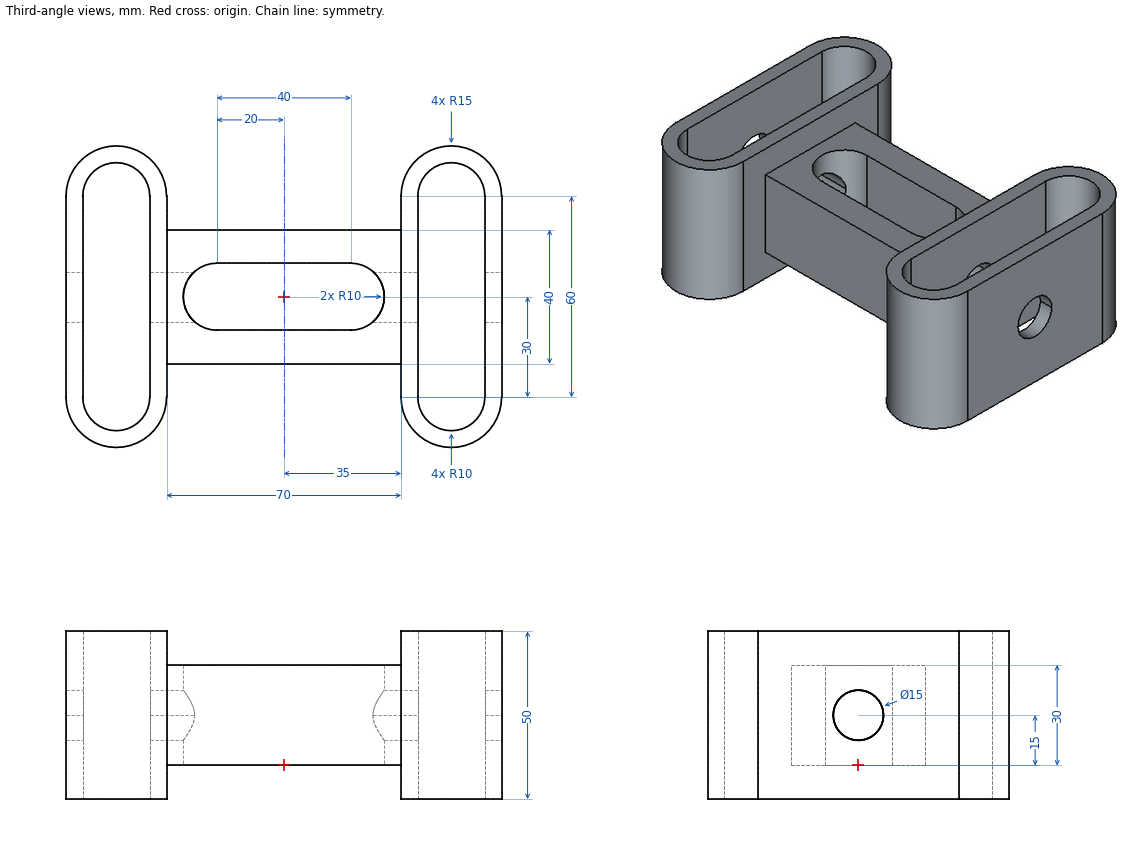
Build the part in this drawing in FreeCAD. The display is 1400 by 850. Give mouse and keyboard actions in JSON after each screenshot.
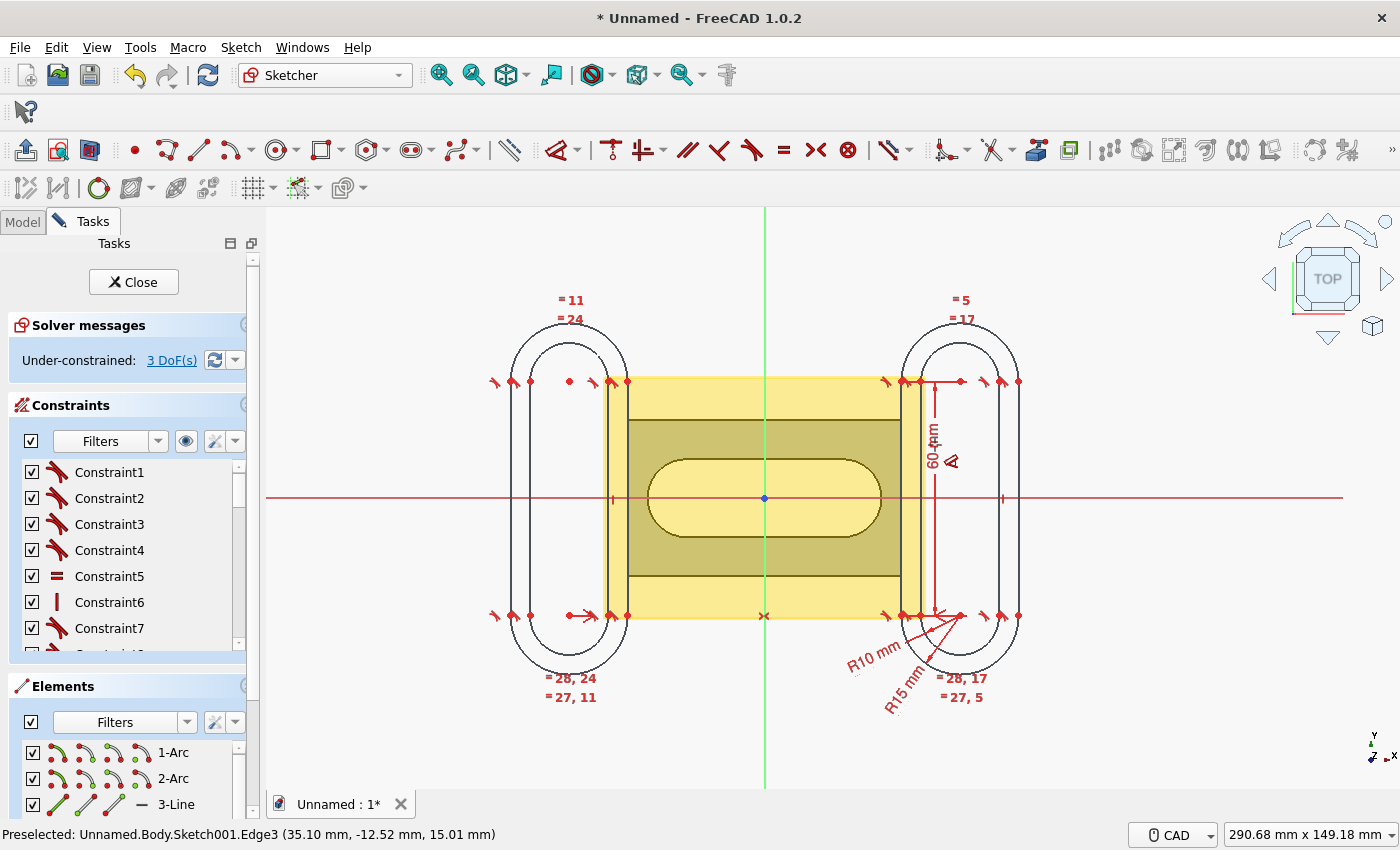
{"action": "left_click", "coordinate": [511, 546]}
{"action": "left_click", "coordinate": [477, 445]}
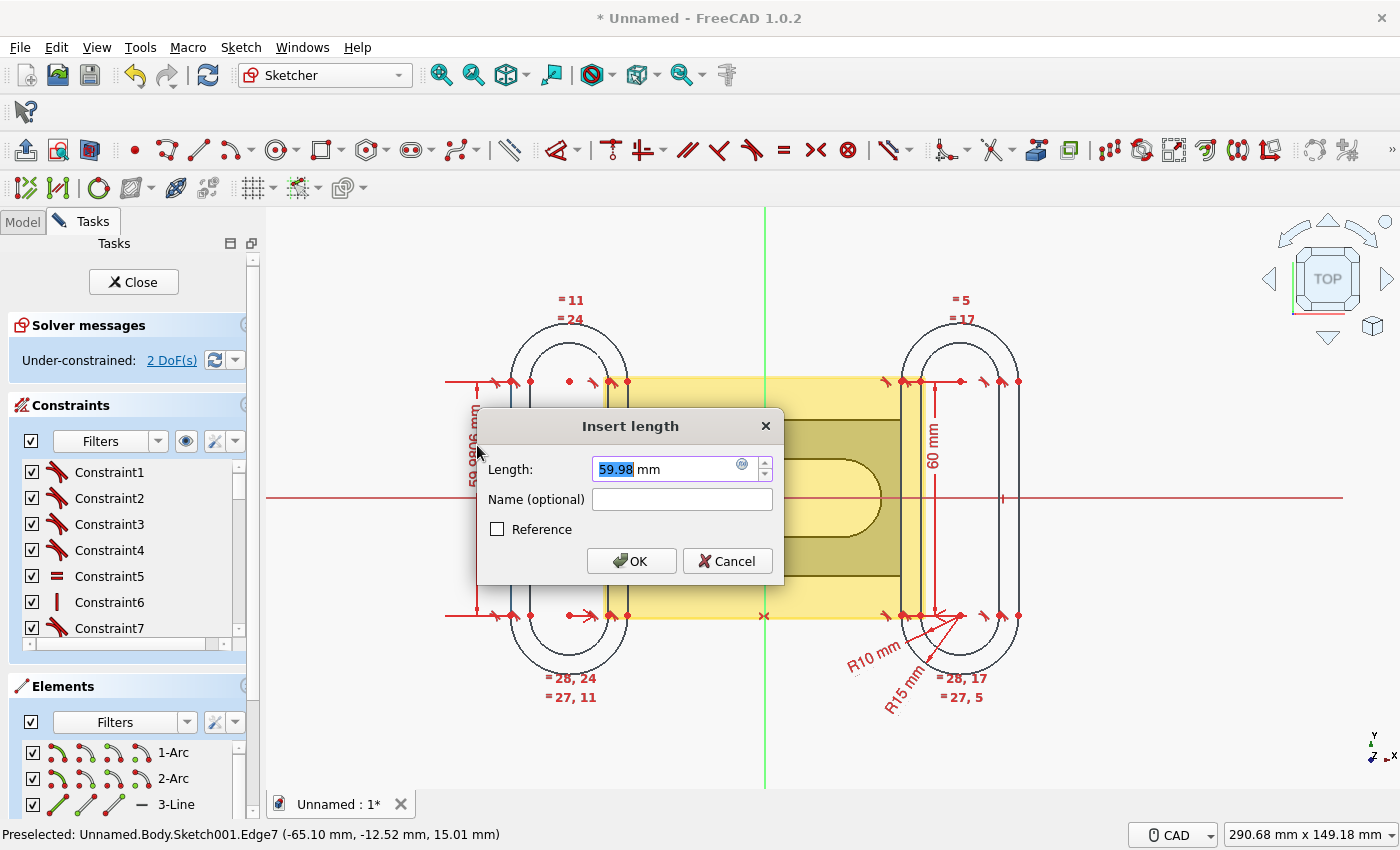
{"action": "type", "text": "60"}
{"action": "key", "text": "Return"}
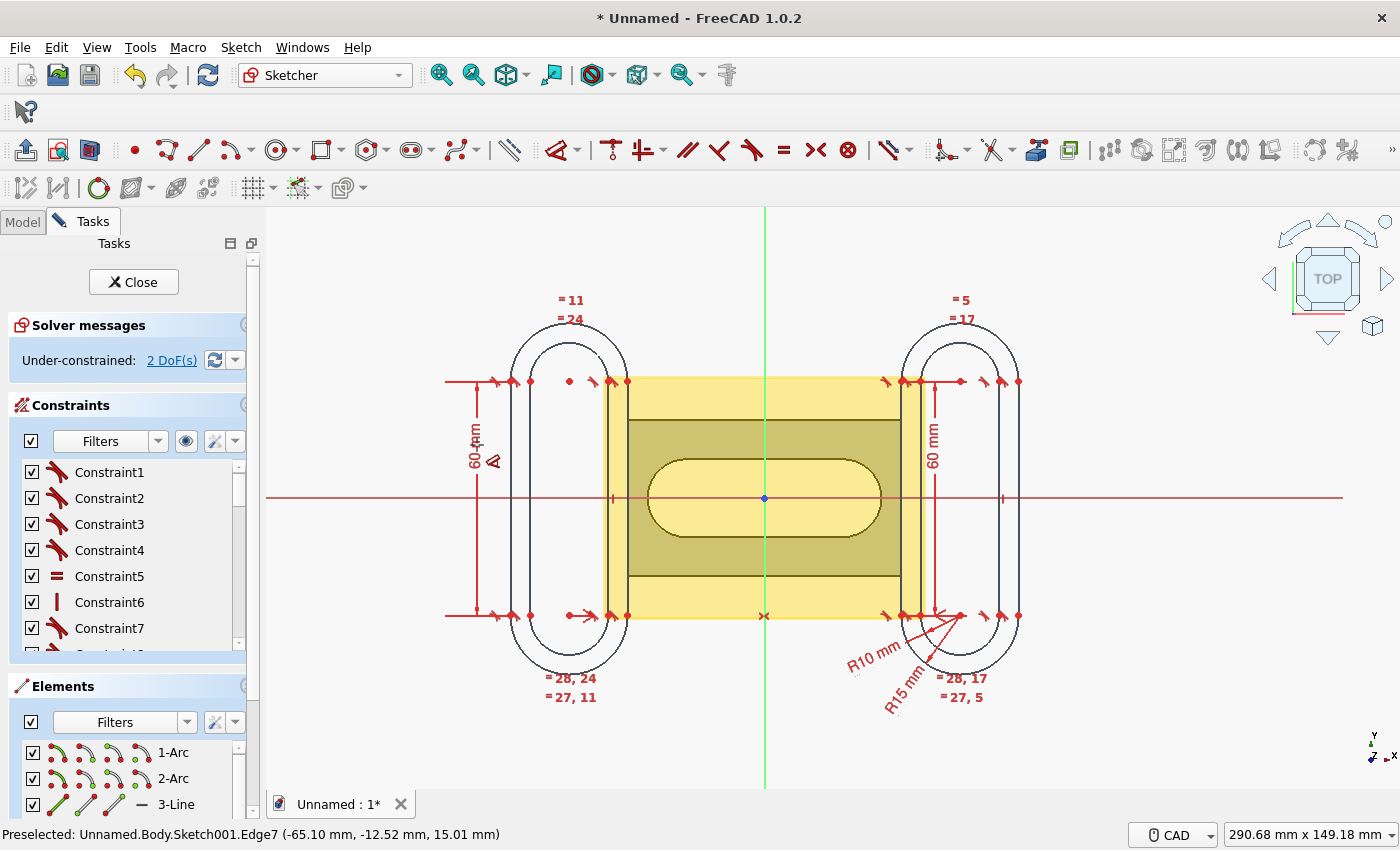
{"action": "left_click", "coordinate": [901, 616]}
{"action": "left_click", "coordinate": [802, 650]}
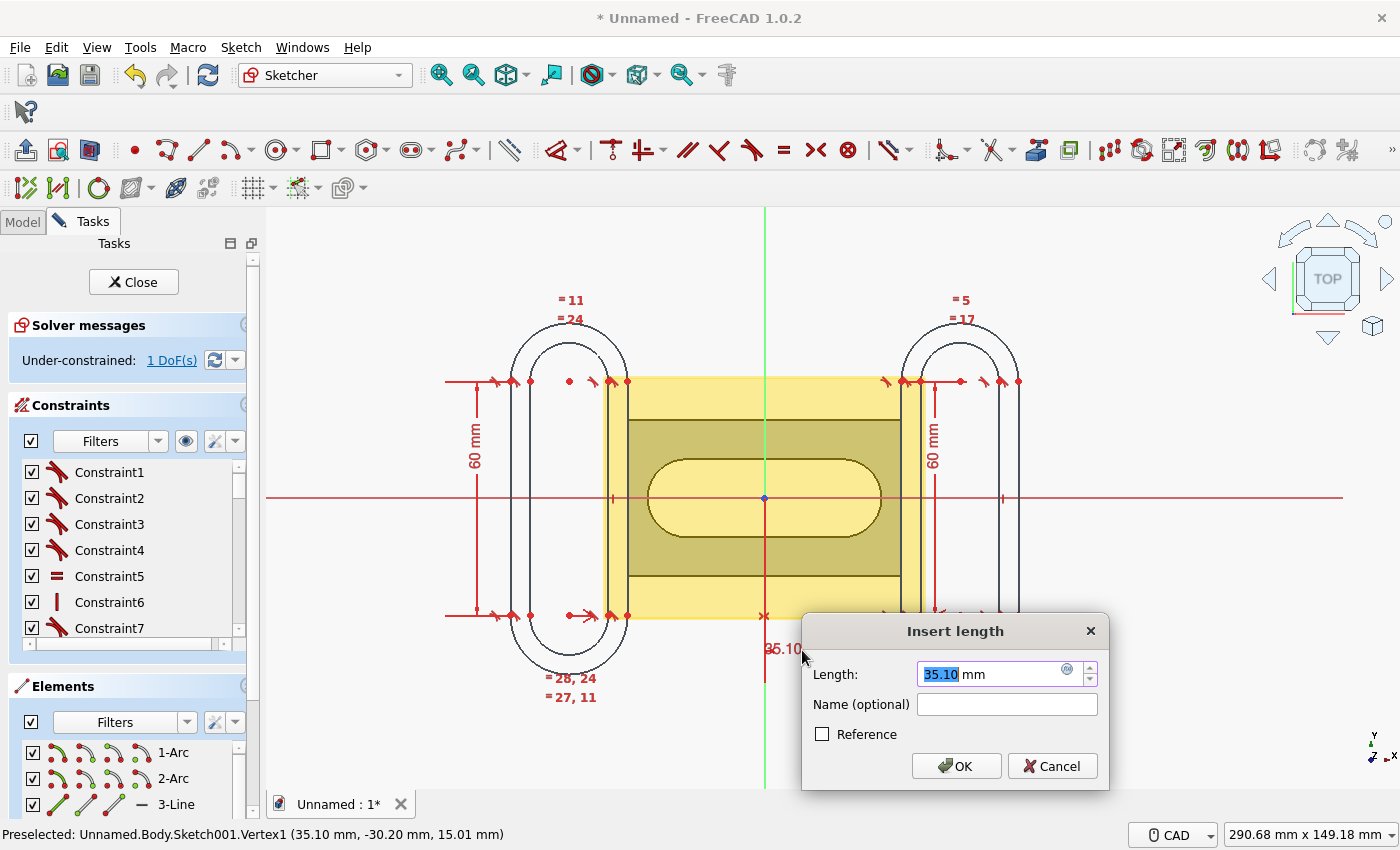
{"action": "type", "text": "35"}
{"action": "key", "text": "Return"}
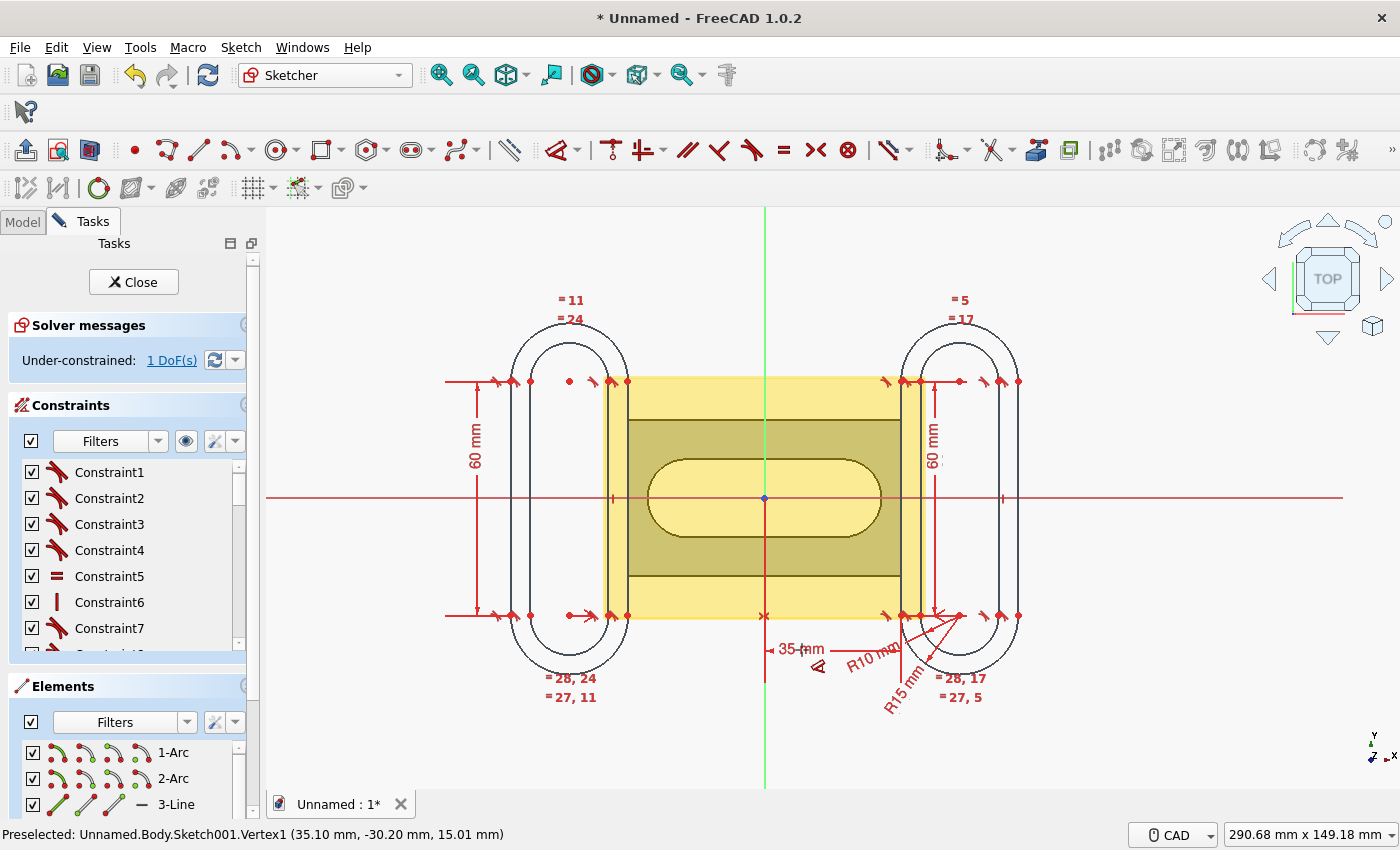
{"action": "left_click", "coordinate": [901, 616]}
{"action": "left_click", "coordinate": [935, 557]}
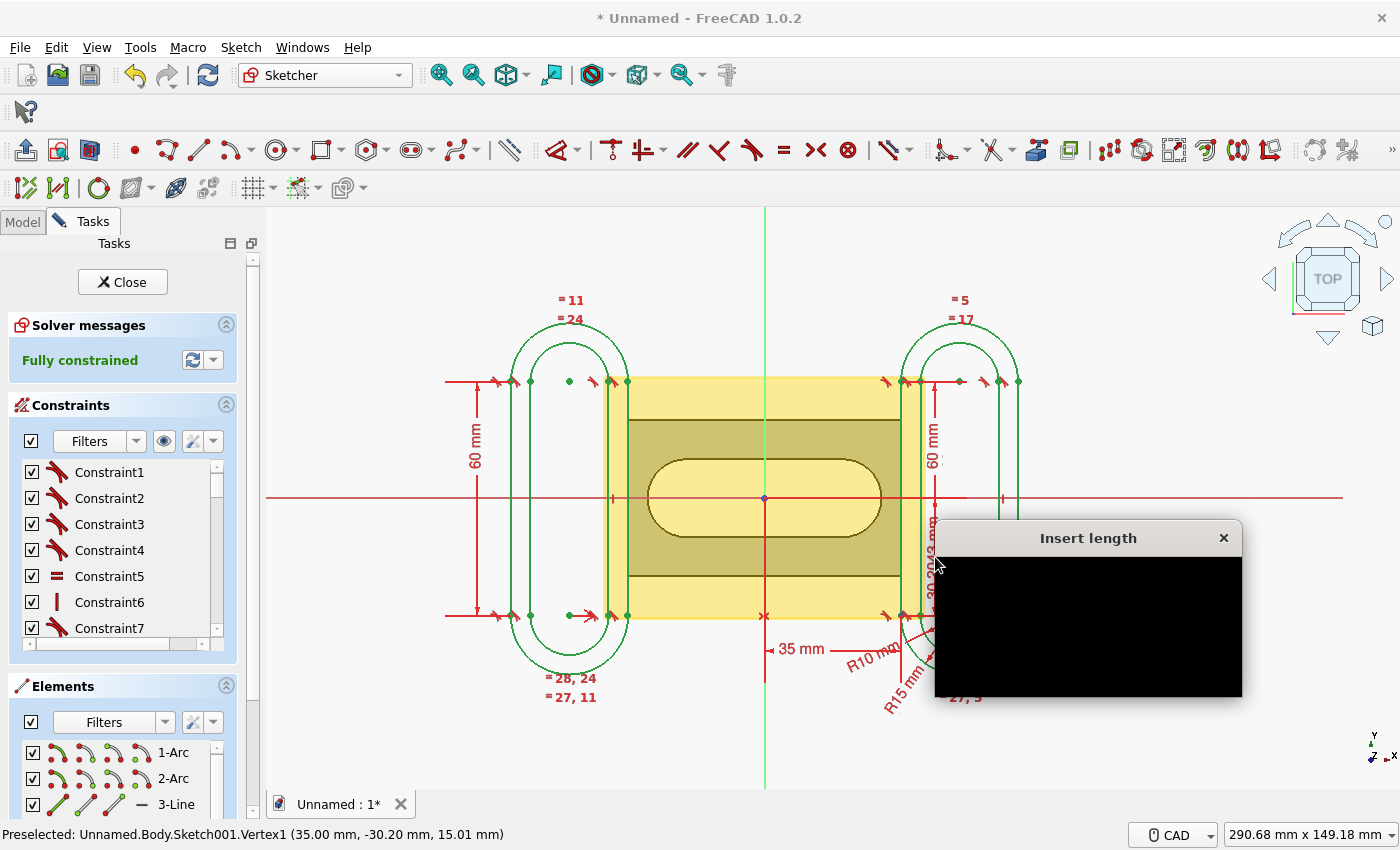
{"action": "type", "text": "30"}
{"action": "key", "text": "Return"}
{"action": "key", "text": "Escape"}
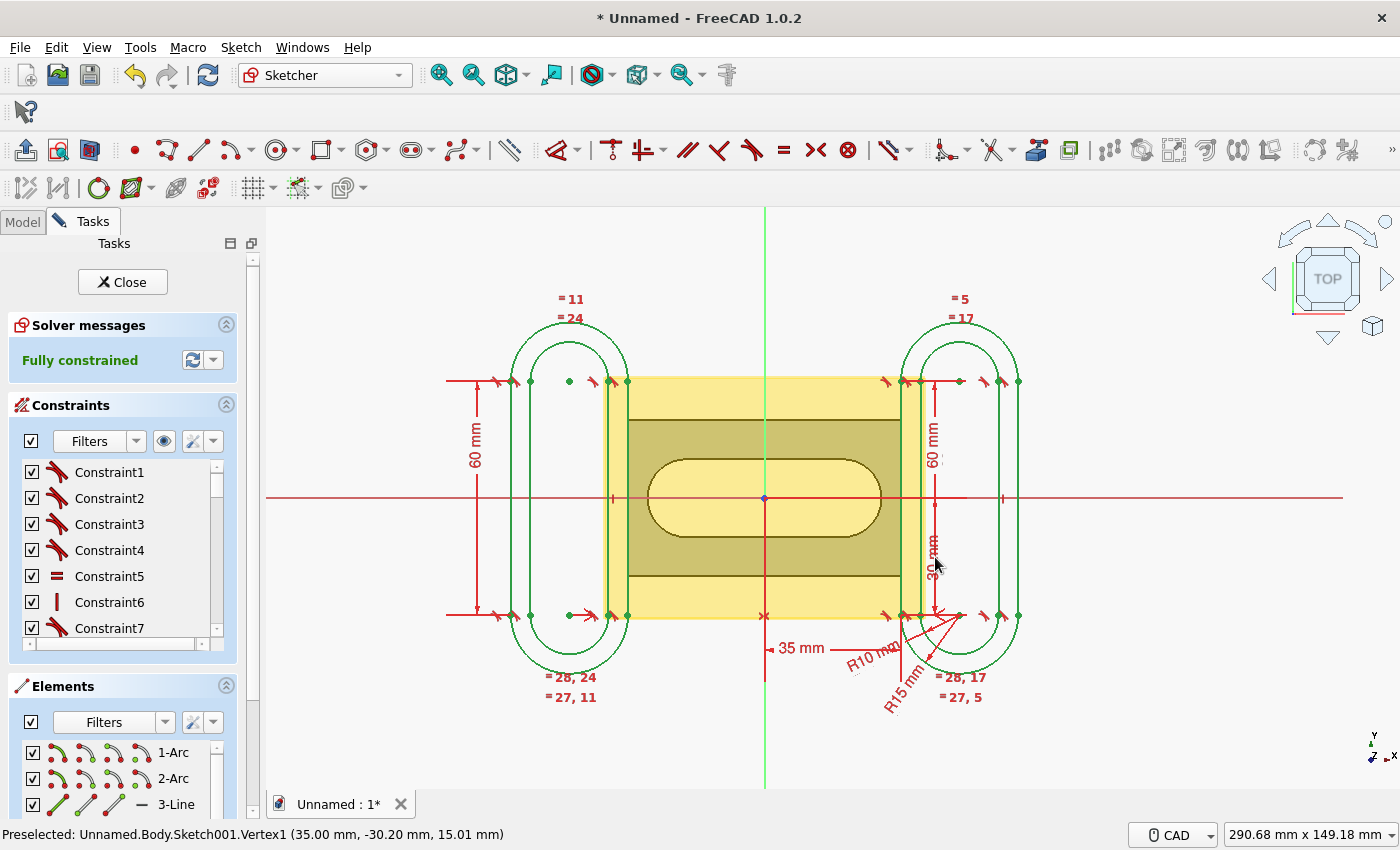
{"action": "left_click", "coordinate": [123, 282]}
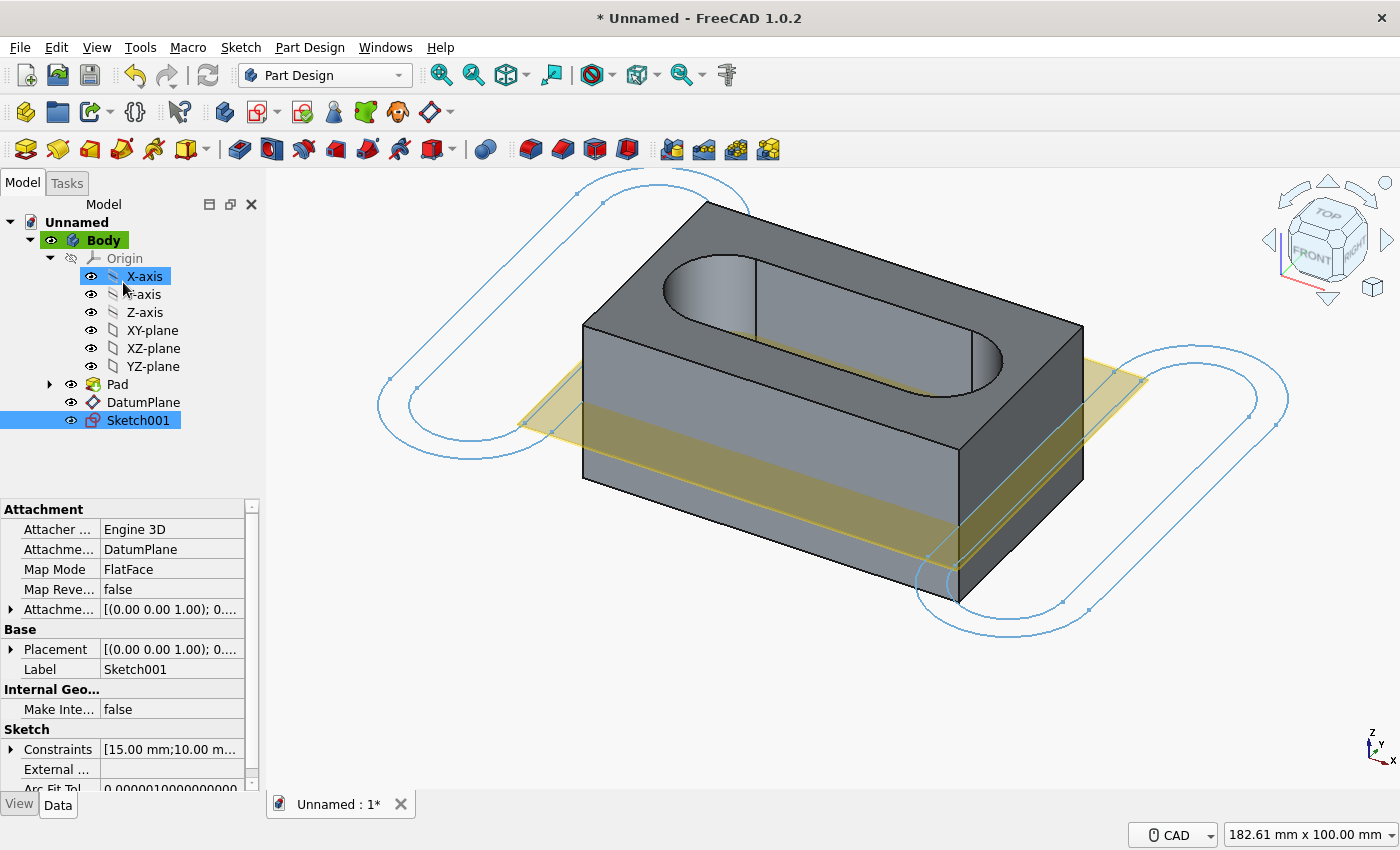
{"action": "left_click", "coordinate": [26, 150]}